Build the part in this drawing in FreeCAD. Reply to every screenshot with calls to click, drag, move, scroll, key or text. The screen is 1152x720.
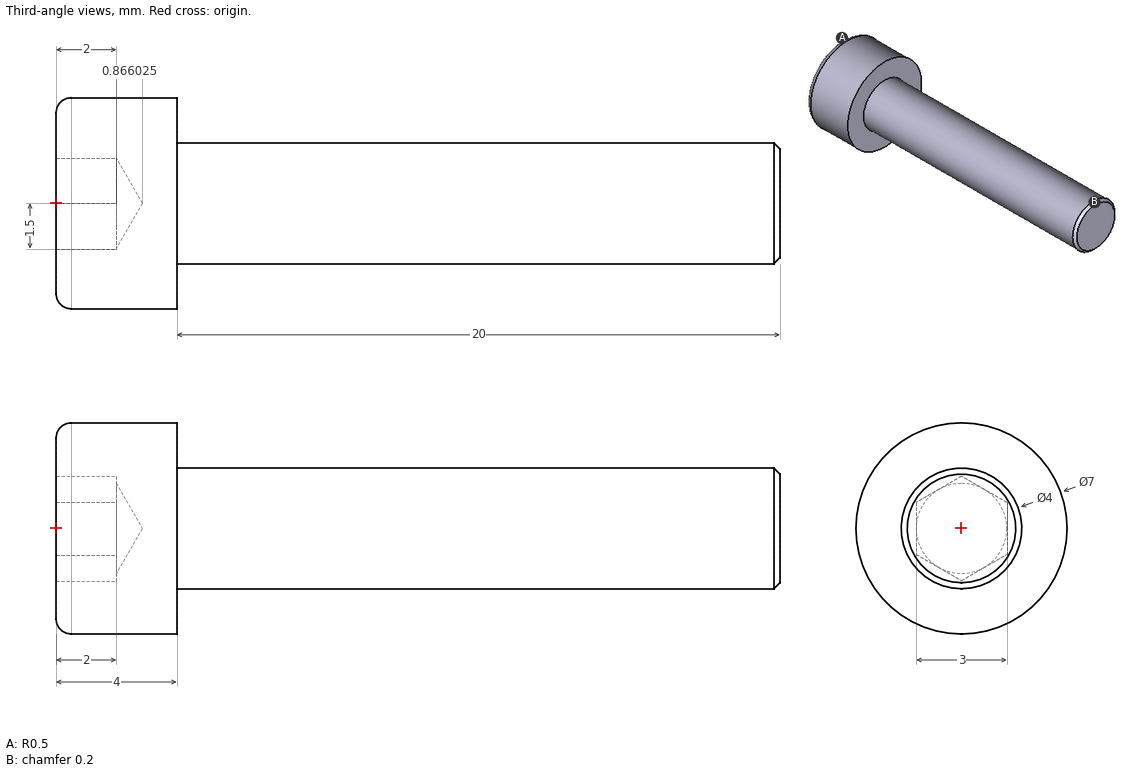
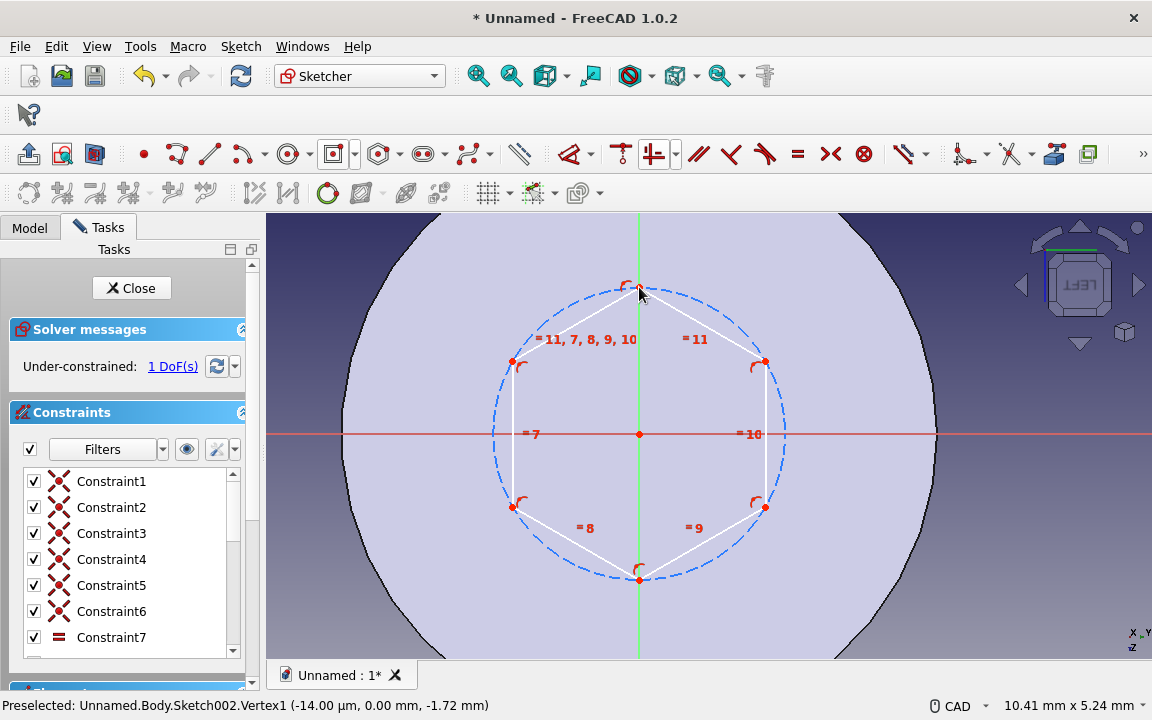
click(568, 154)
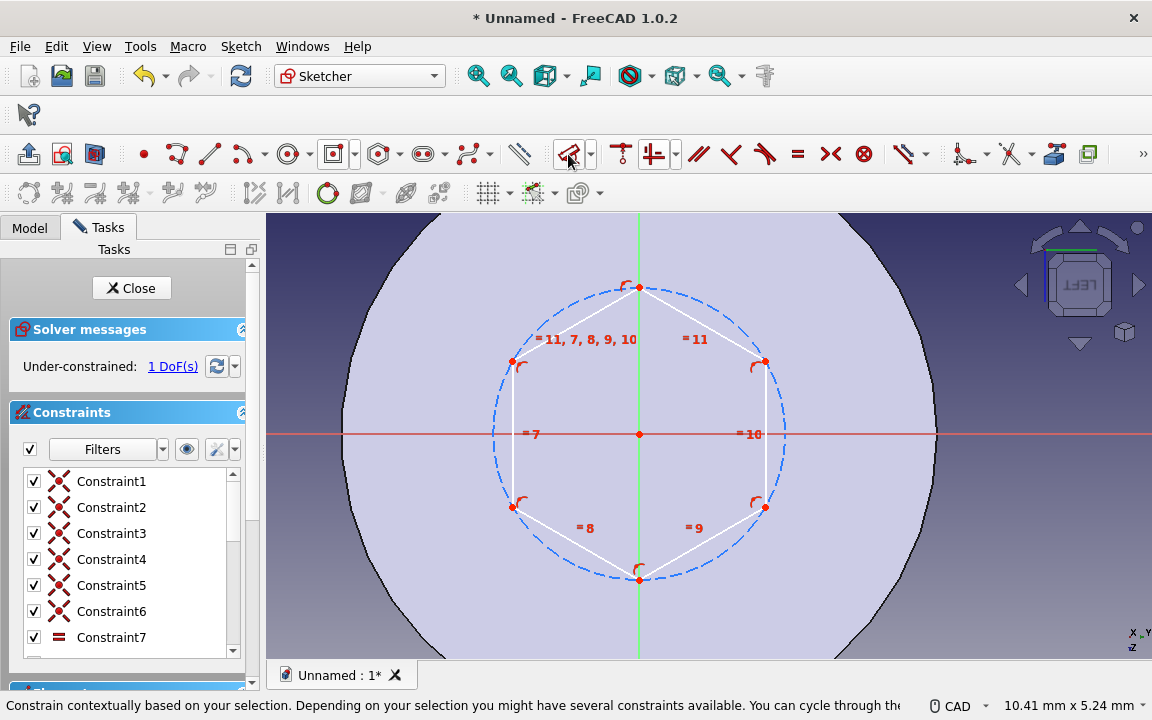
click(513, 361)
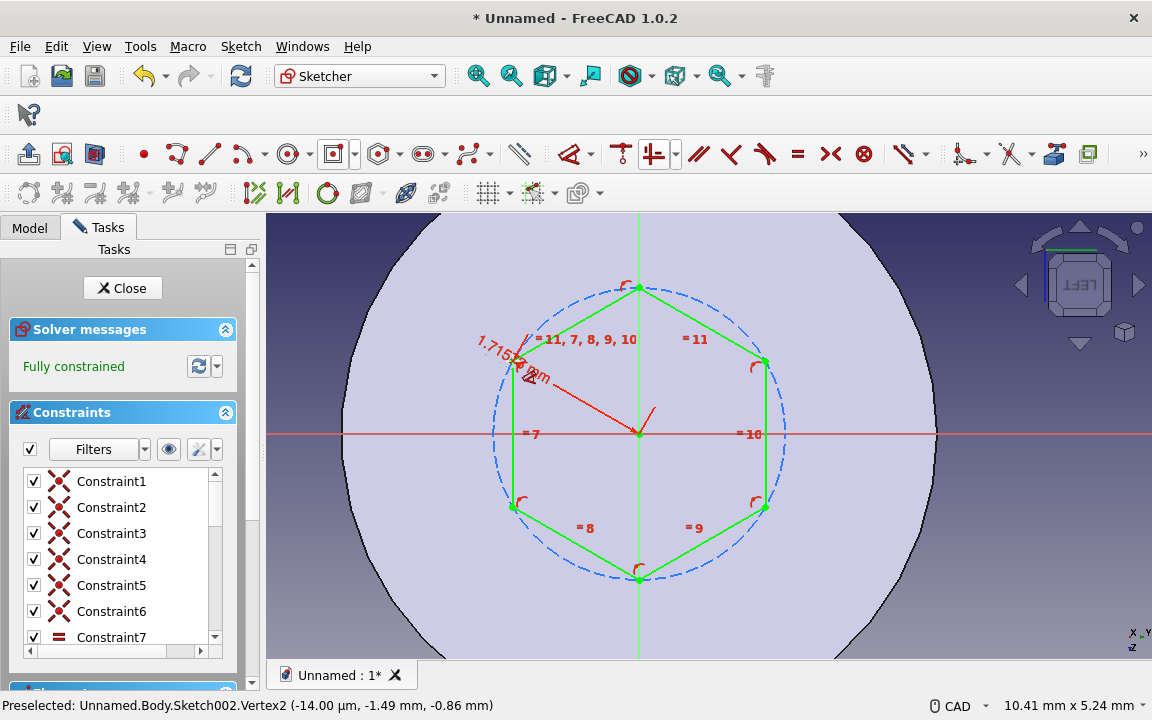
click(766, 507)
click(581, 589)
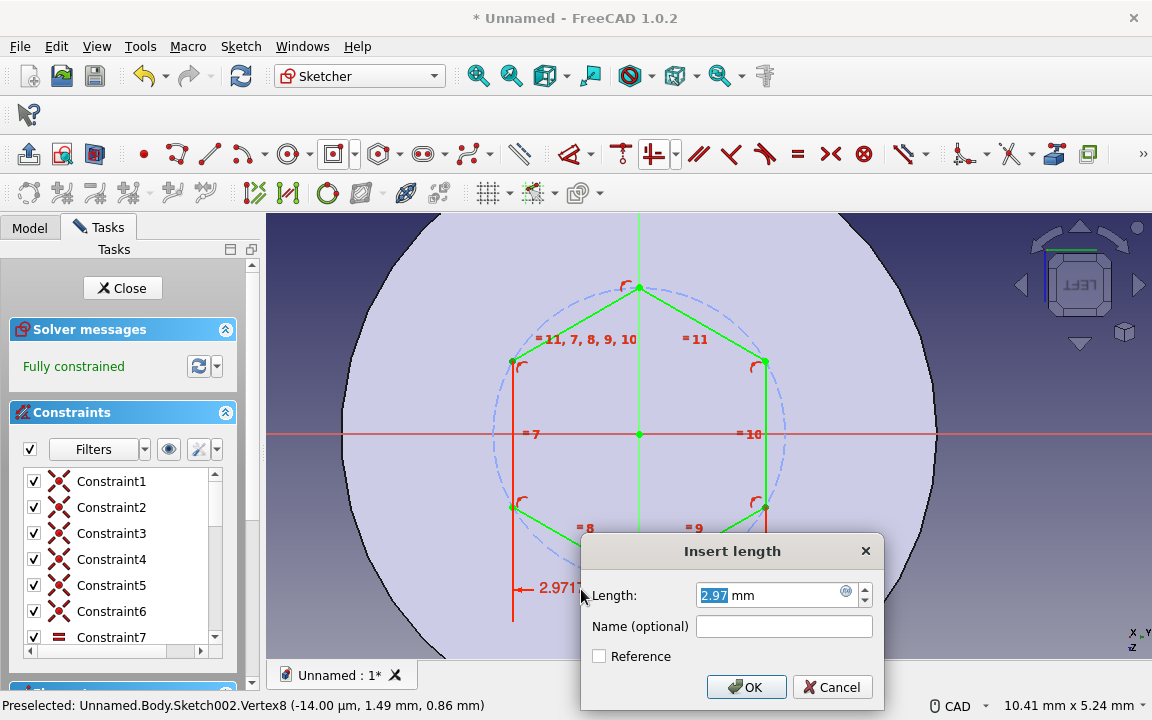
text(3)
key(Return)
key(Escape)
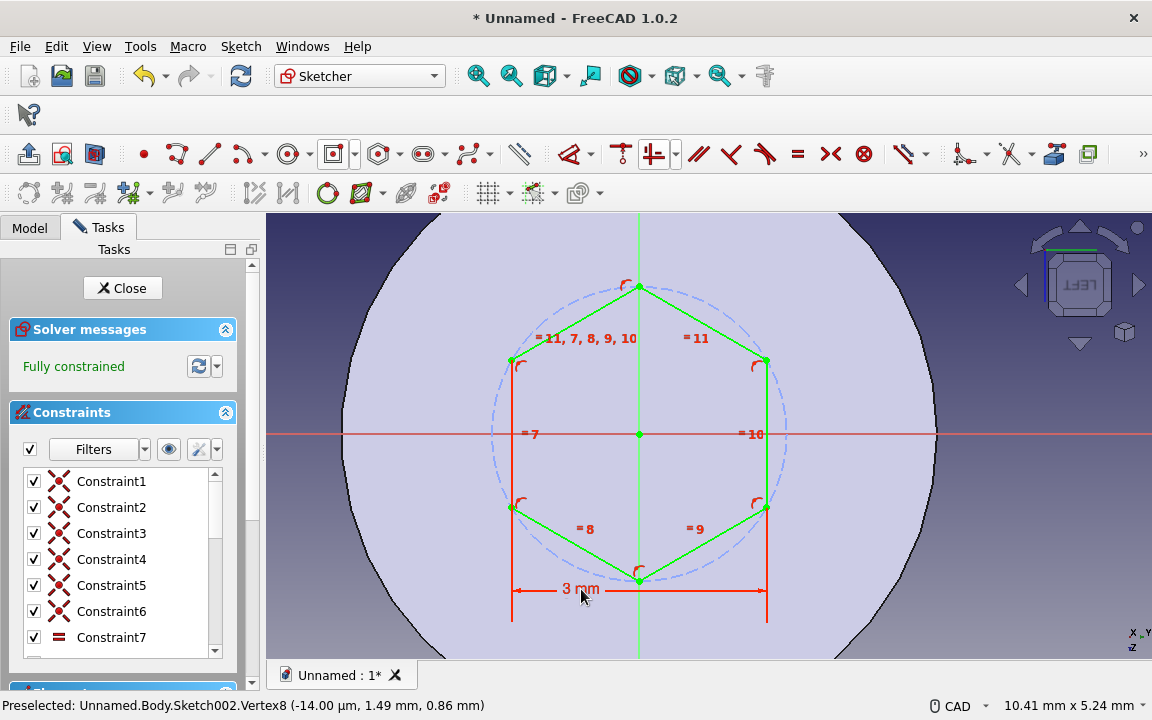
click(123, 288)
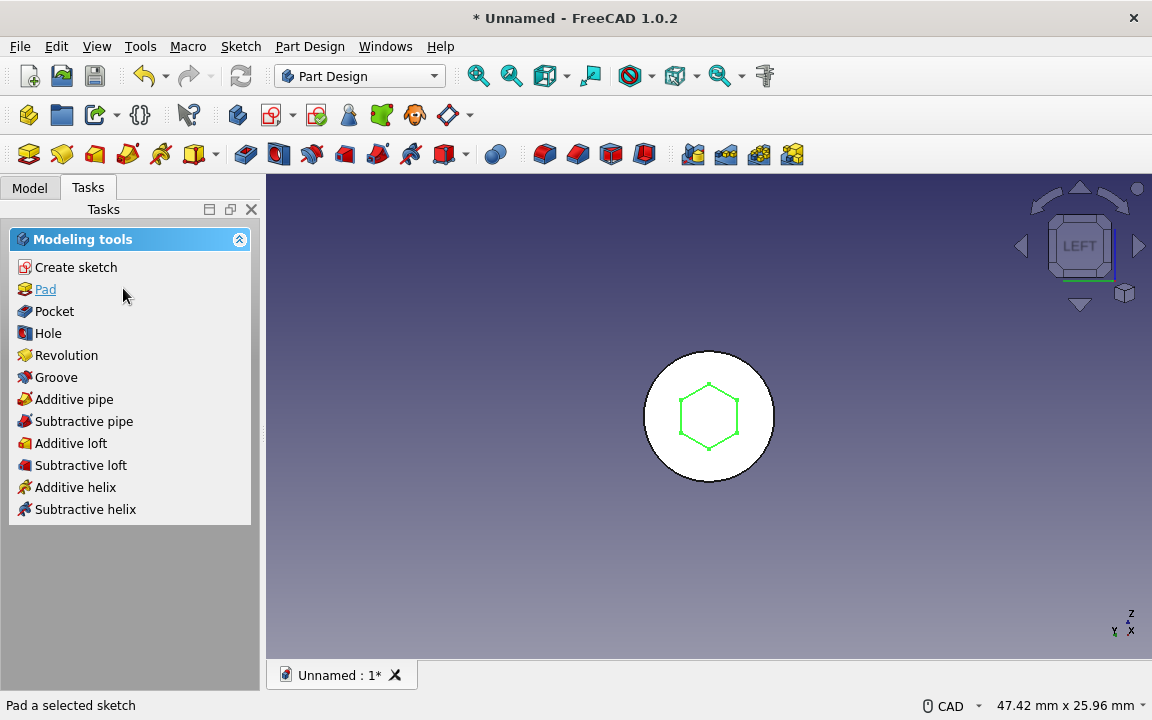
click(246, 154)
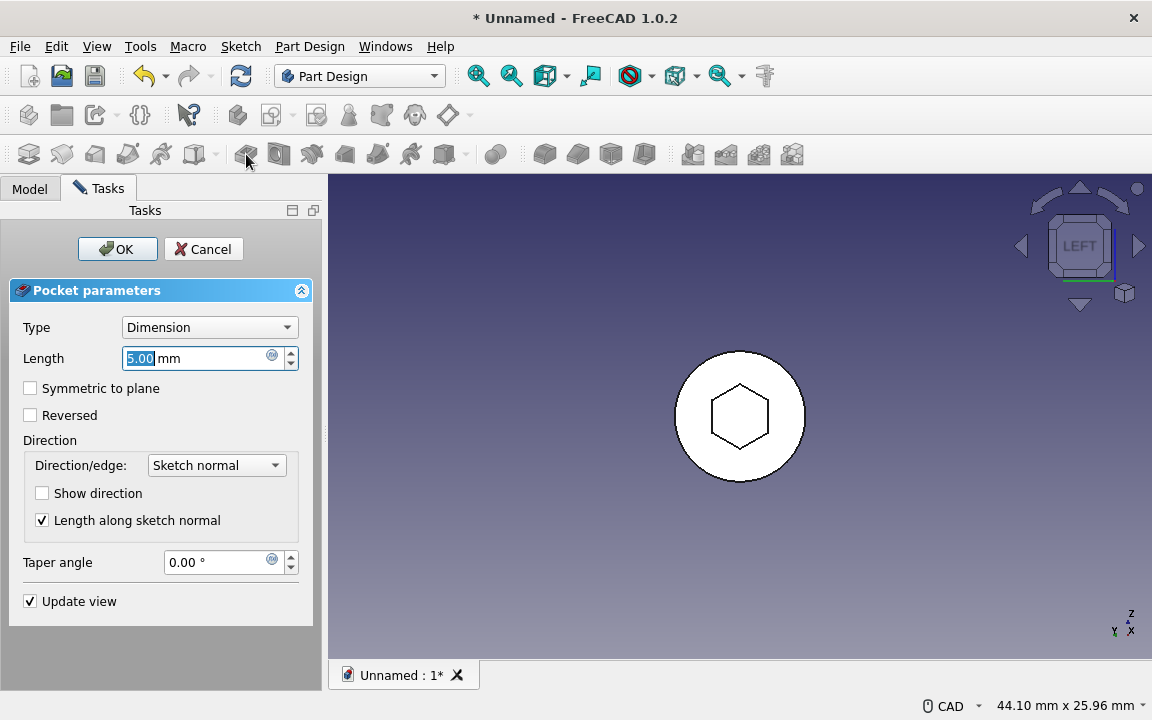
text(2)
key(Tab)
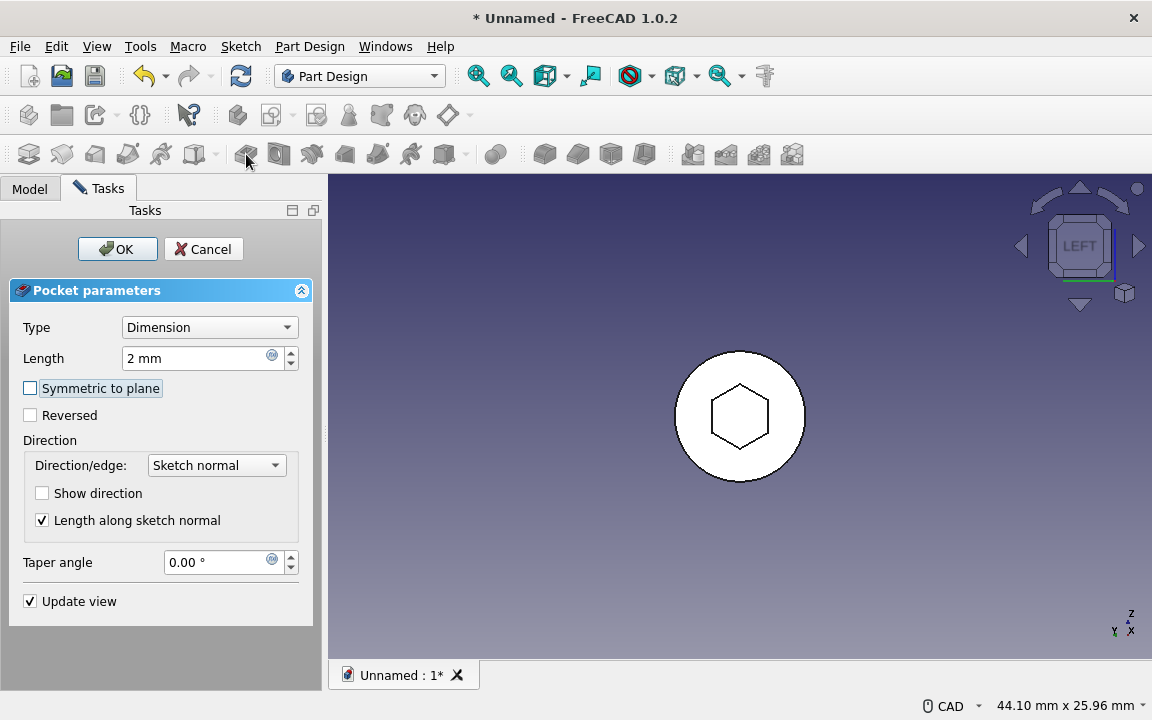
click(118, 249)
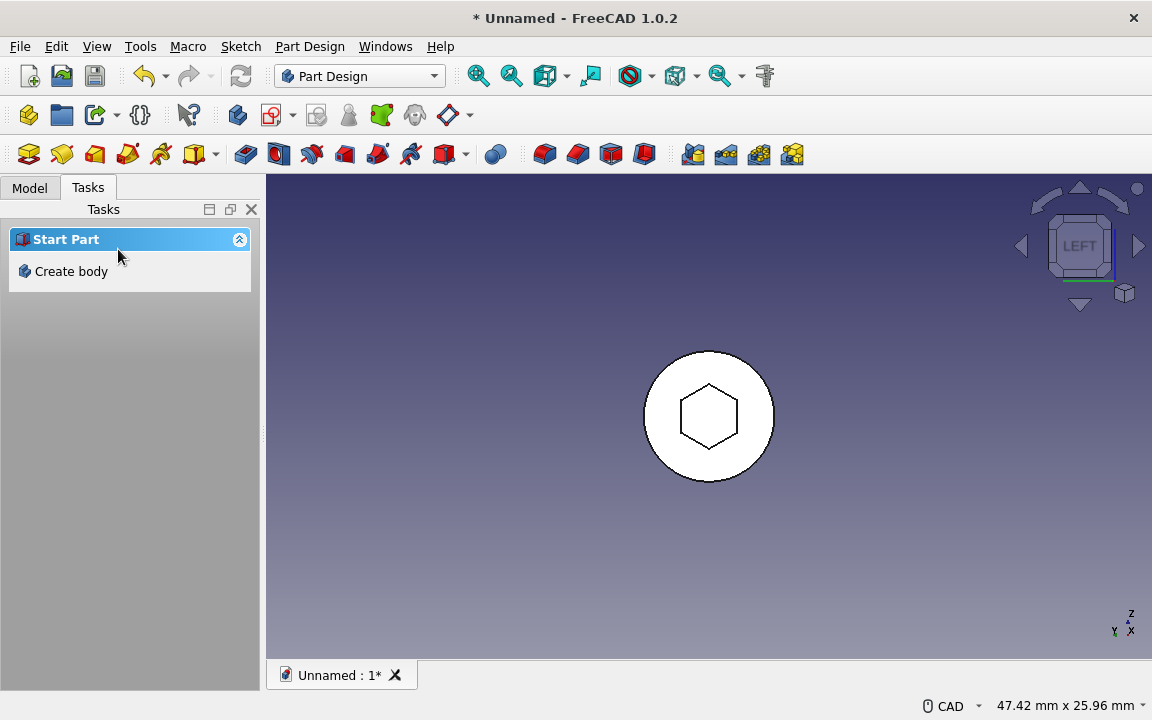
click(479, 76)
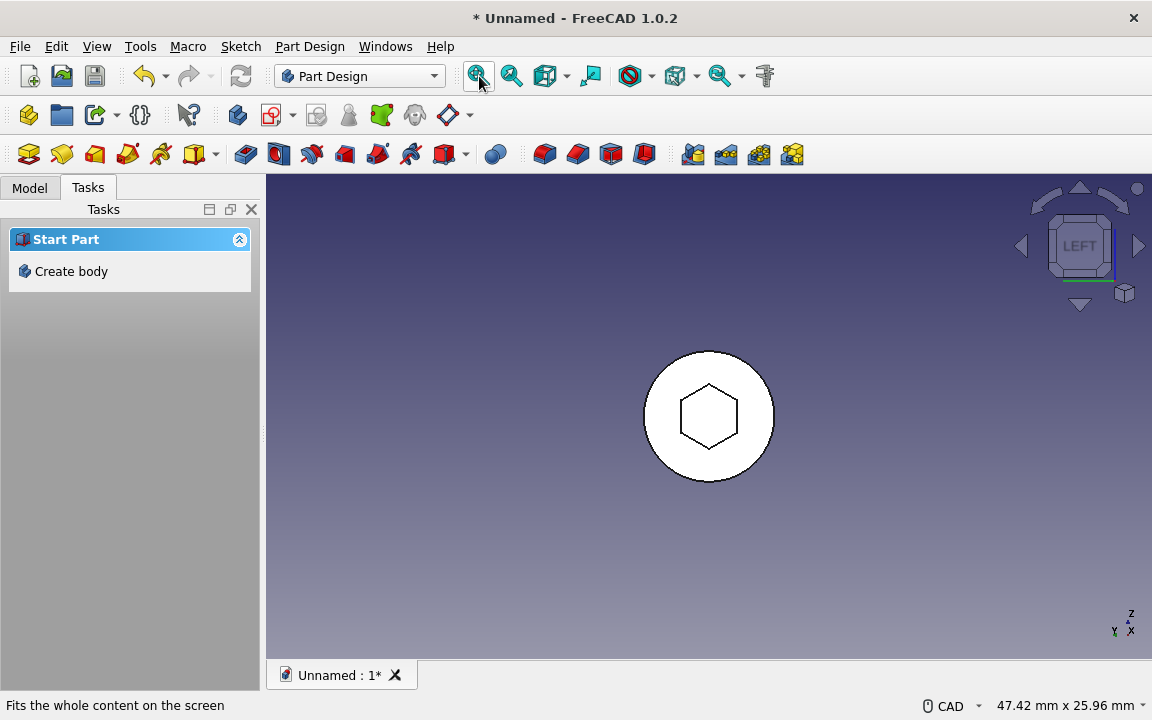
click(270, 116)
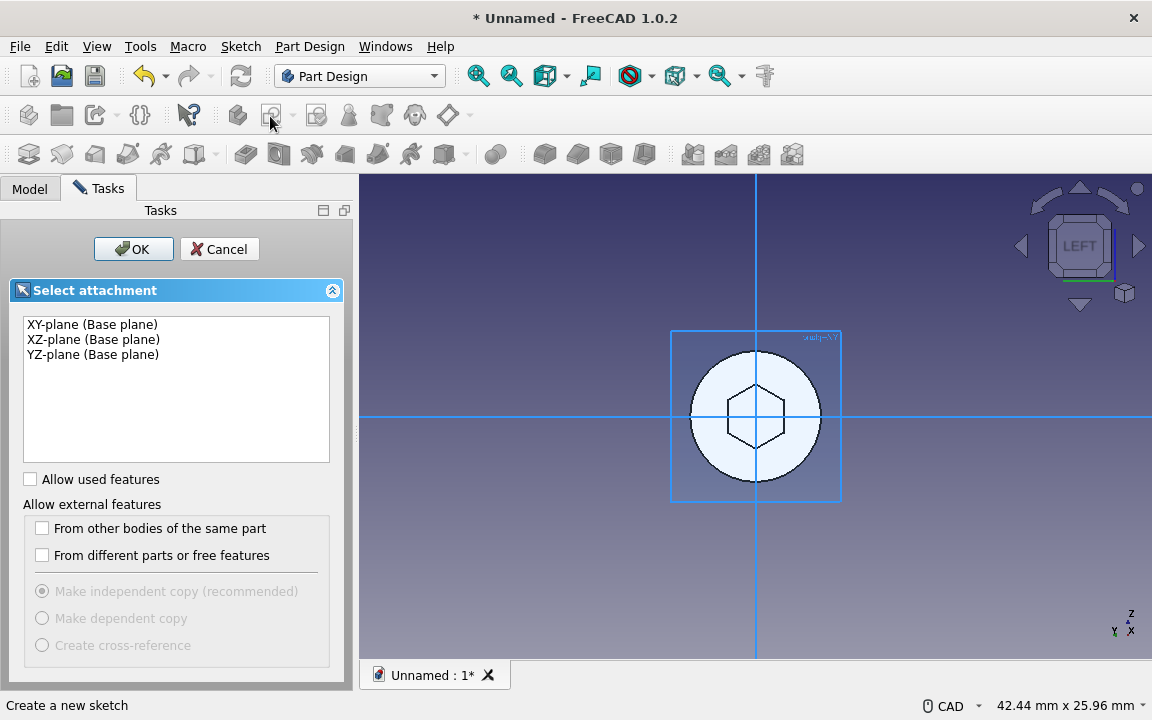
click(84, 324)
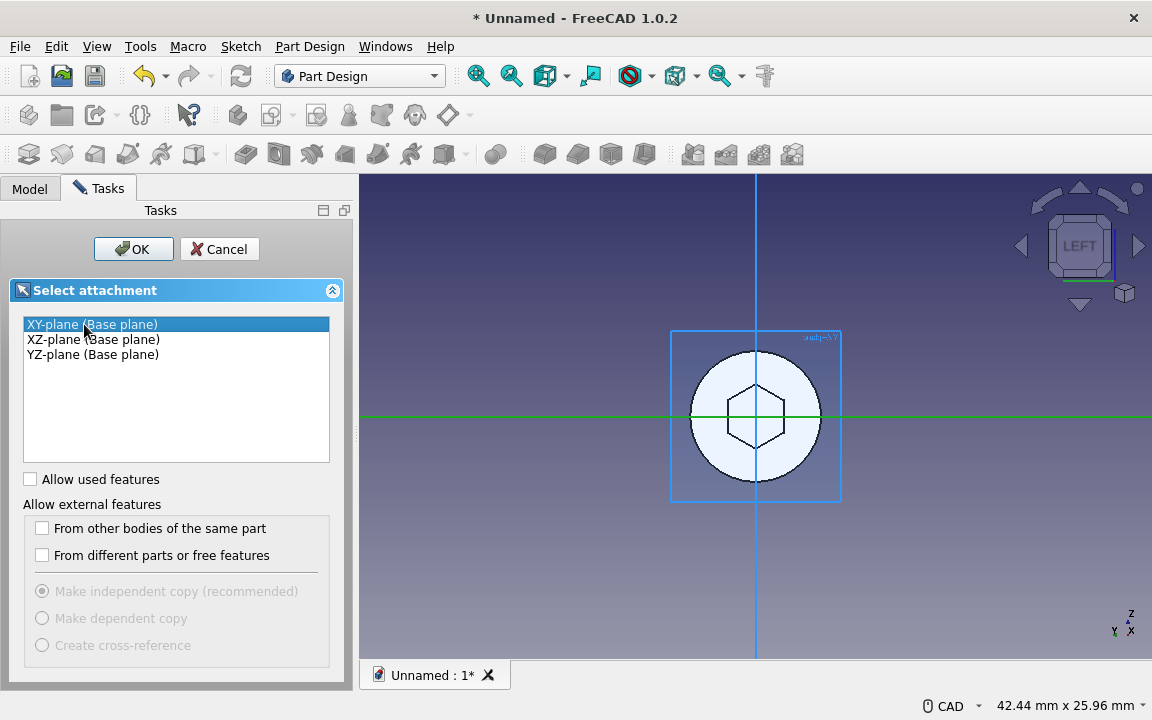
click(134, 249)